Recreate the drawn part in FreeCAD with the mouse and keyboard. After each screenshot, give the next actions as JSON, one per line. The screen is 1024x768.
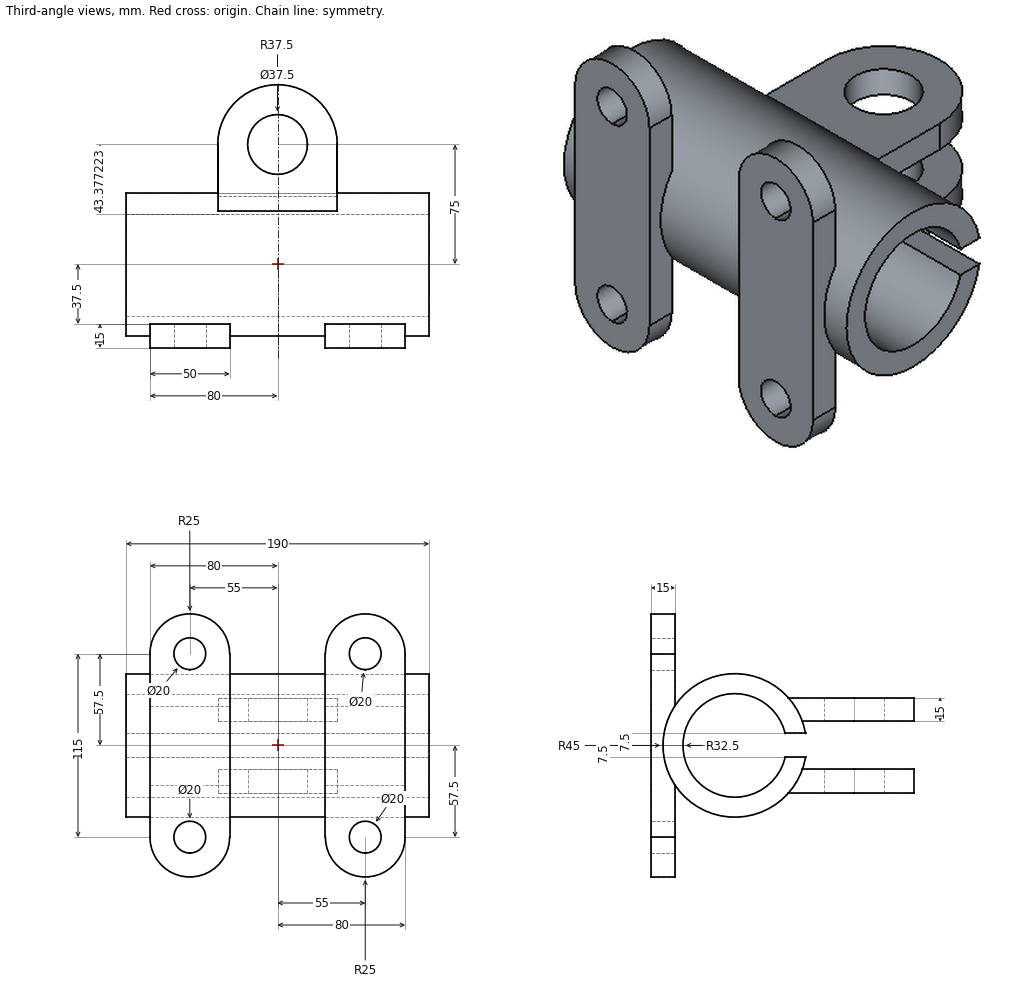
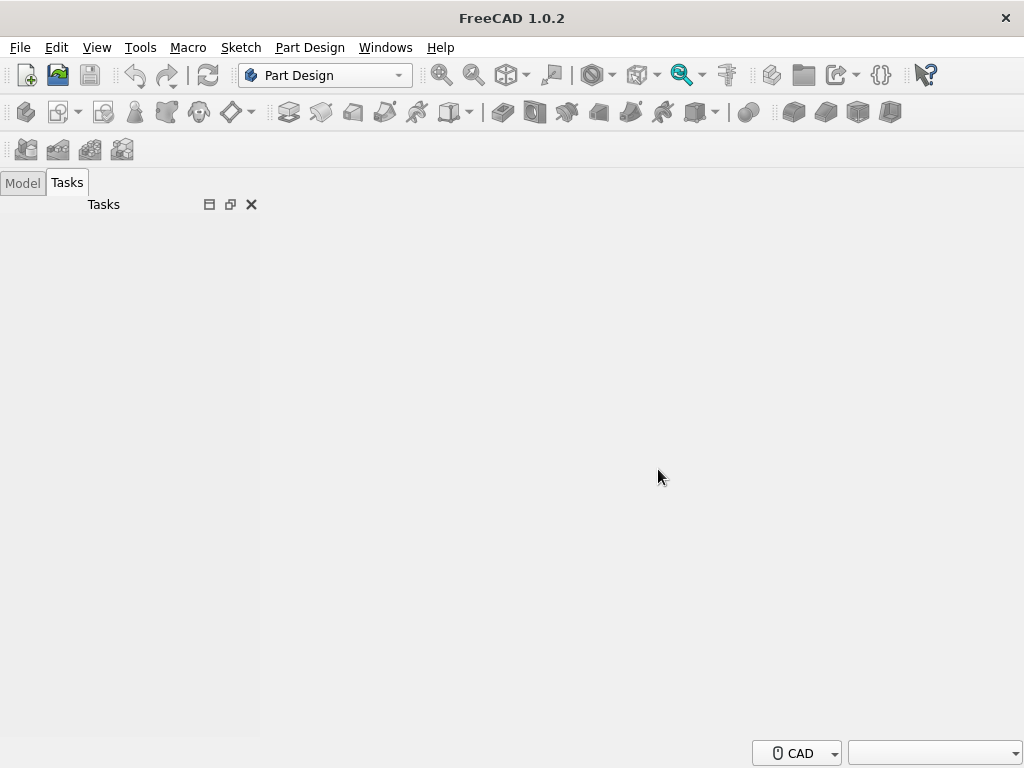
{"action": "left_click", "coordinate": [26, 76]}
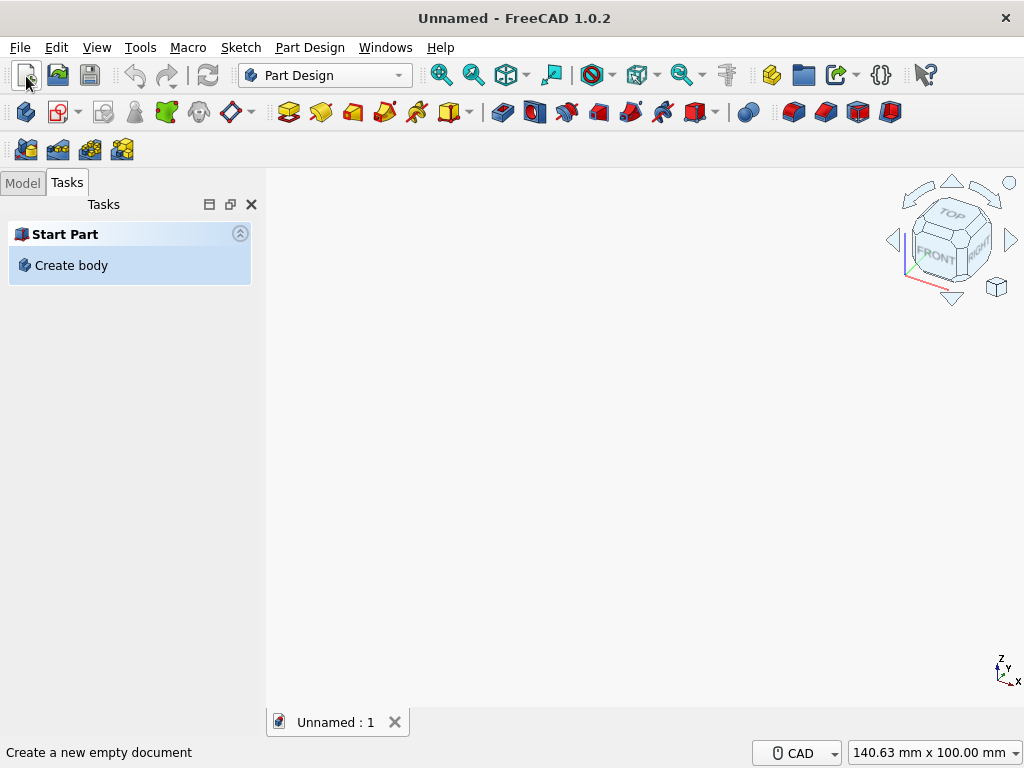
{"action": "left_click", "coordinate": [58, 112]}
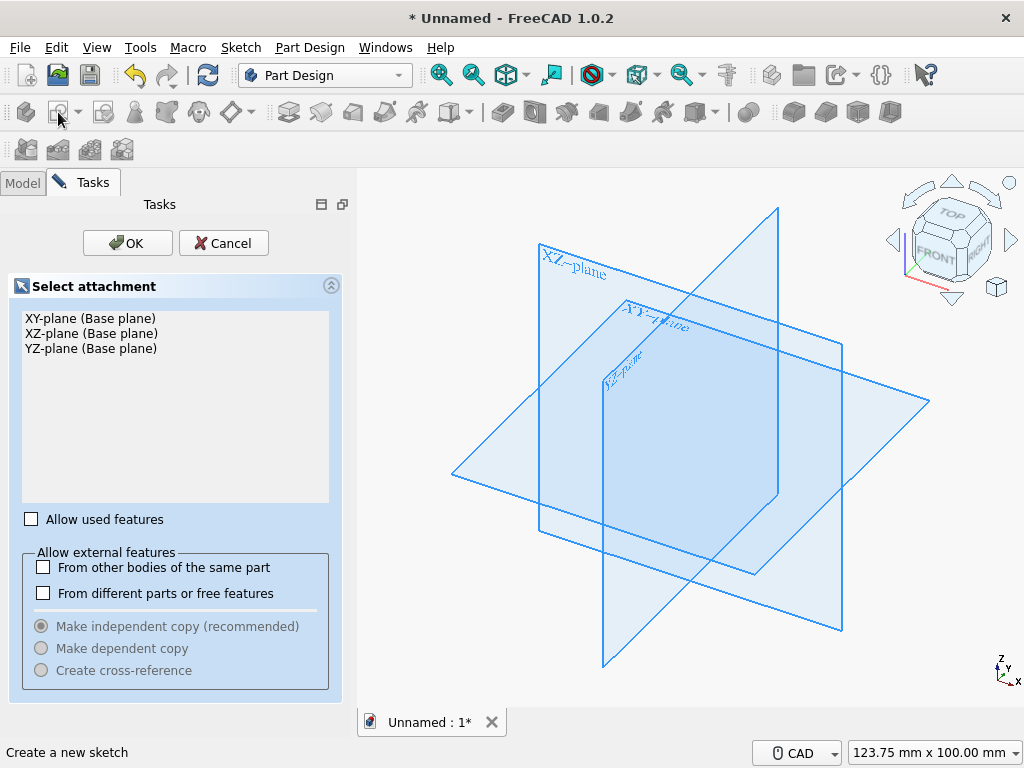
{"action": "left_click", "coordinate": [82, 348]}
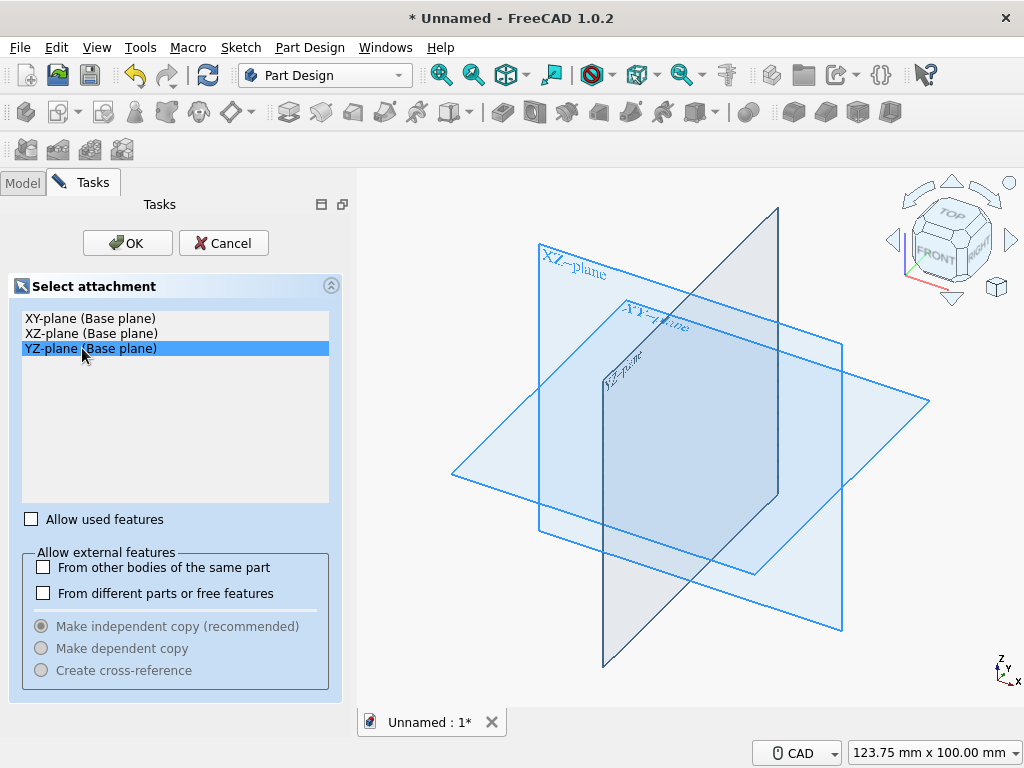
{"action": "left_click", "coordinate": [128, 243]}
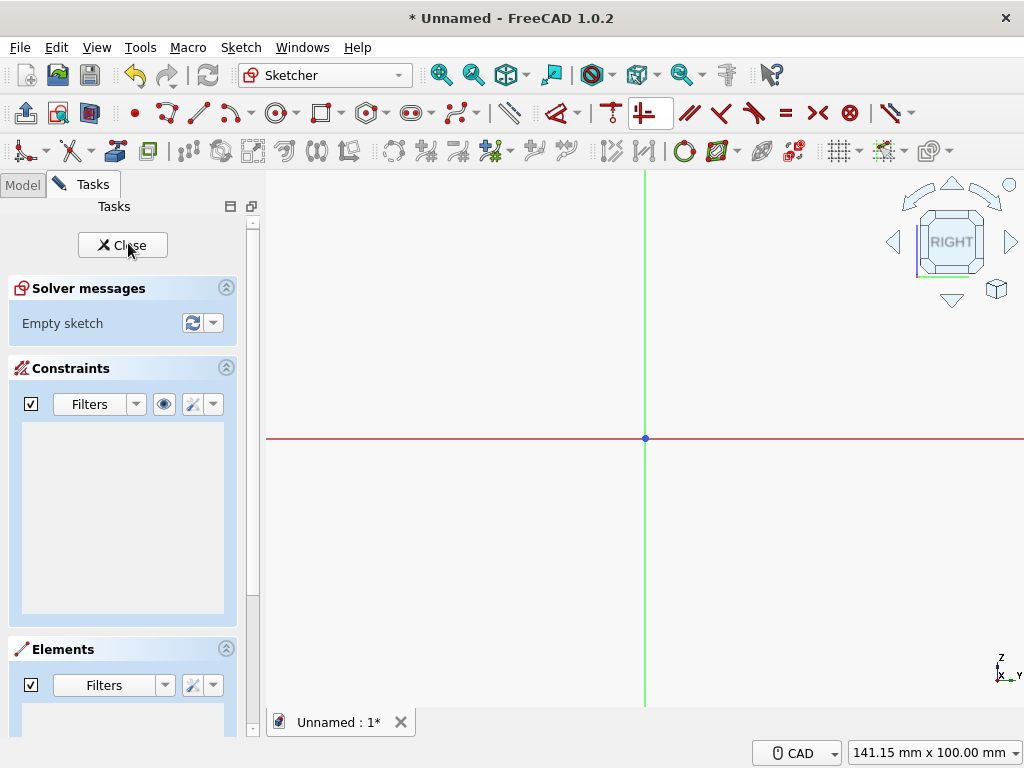
{"action": "scroll", "coordinate": [294, 439], "scroll_direction": "down", "scroll_amount": 1}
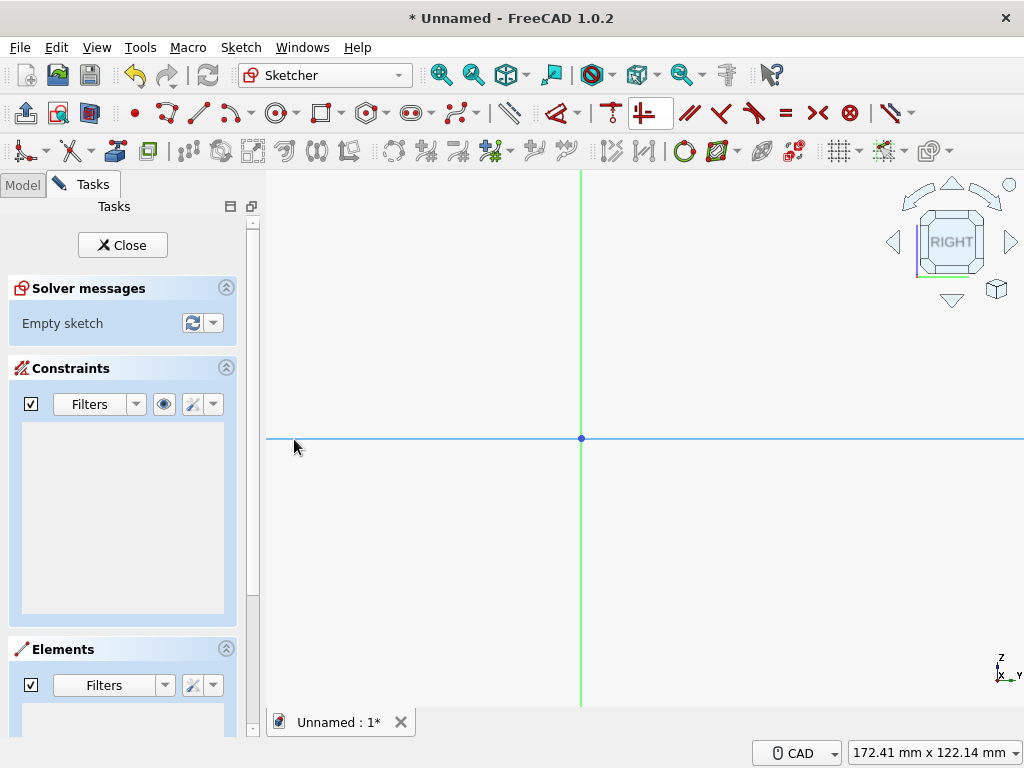
{"action": "left_click", "coordinate": [200, 114]}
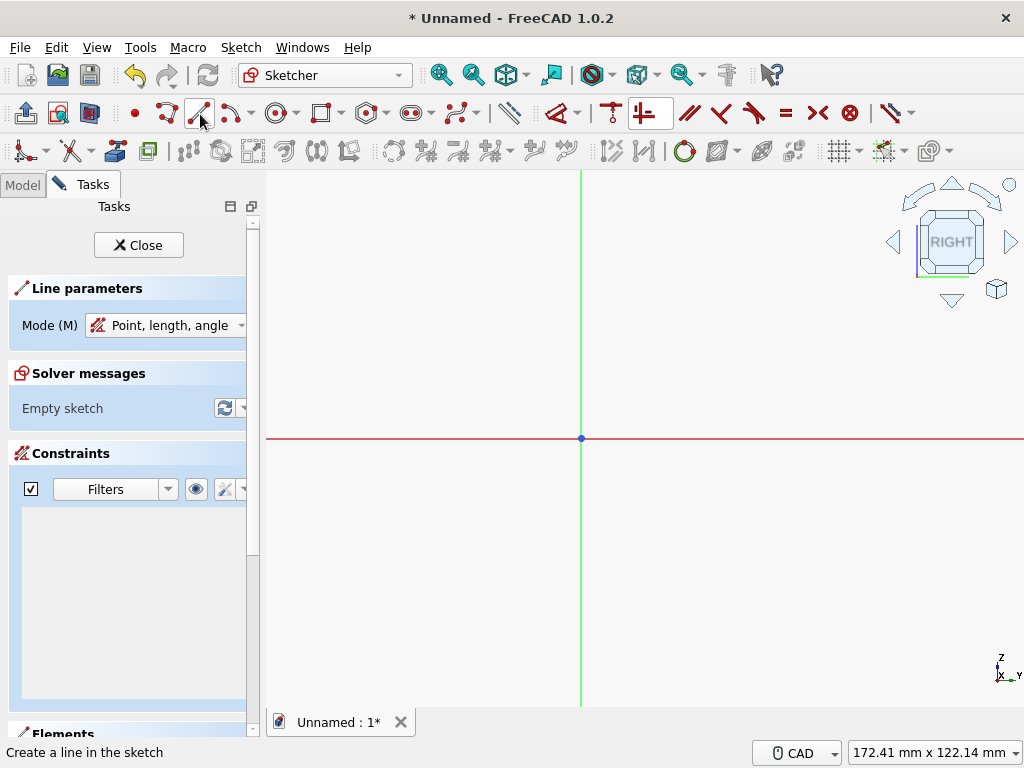
{"action": "left_click", "coordinate": [720, 406]}
{"action": "left_click", "coordinate": [776, 406]}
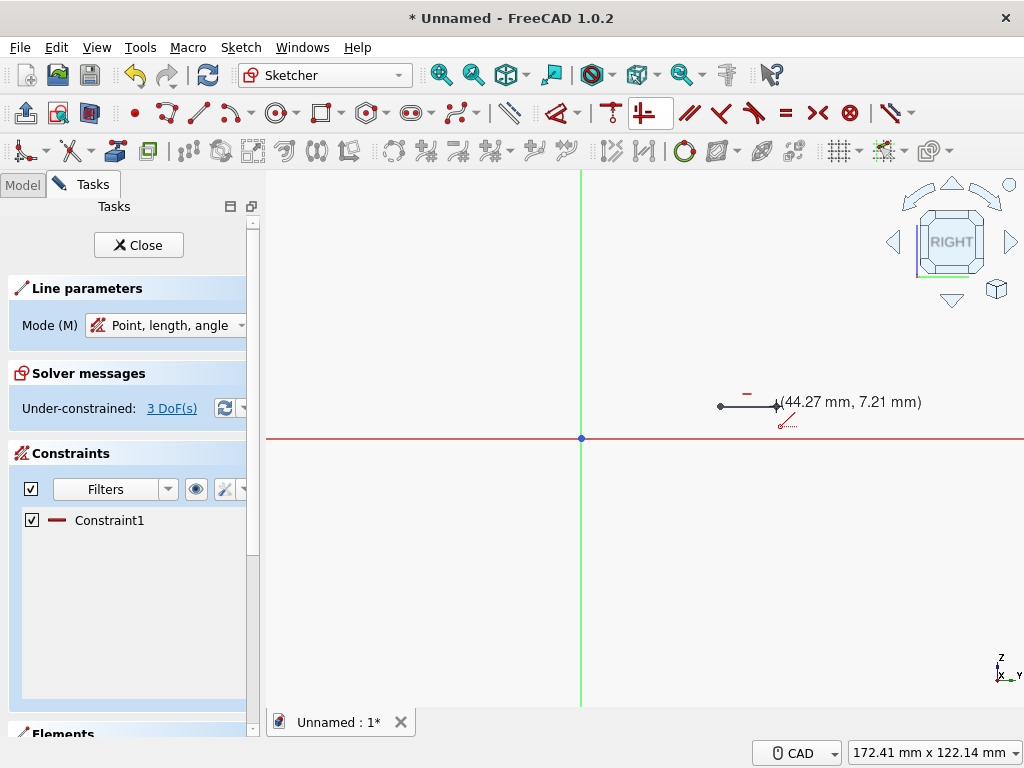
{"action": "left_click", "coordinate": [776, 472]}
{"action": "left_click", "coordinate": [720, 472]}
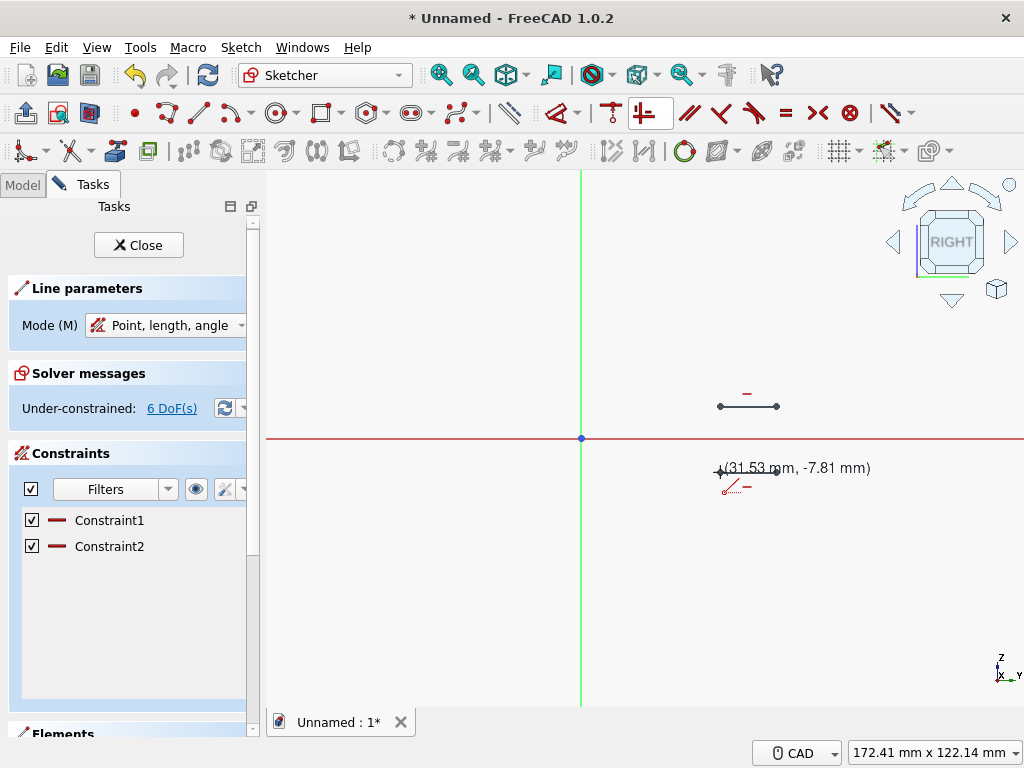
{"action": "left_click", "coordinate": [254, 114]}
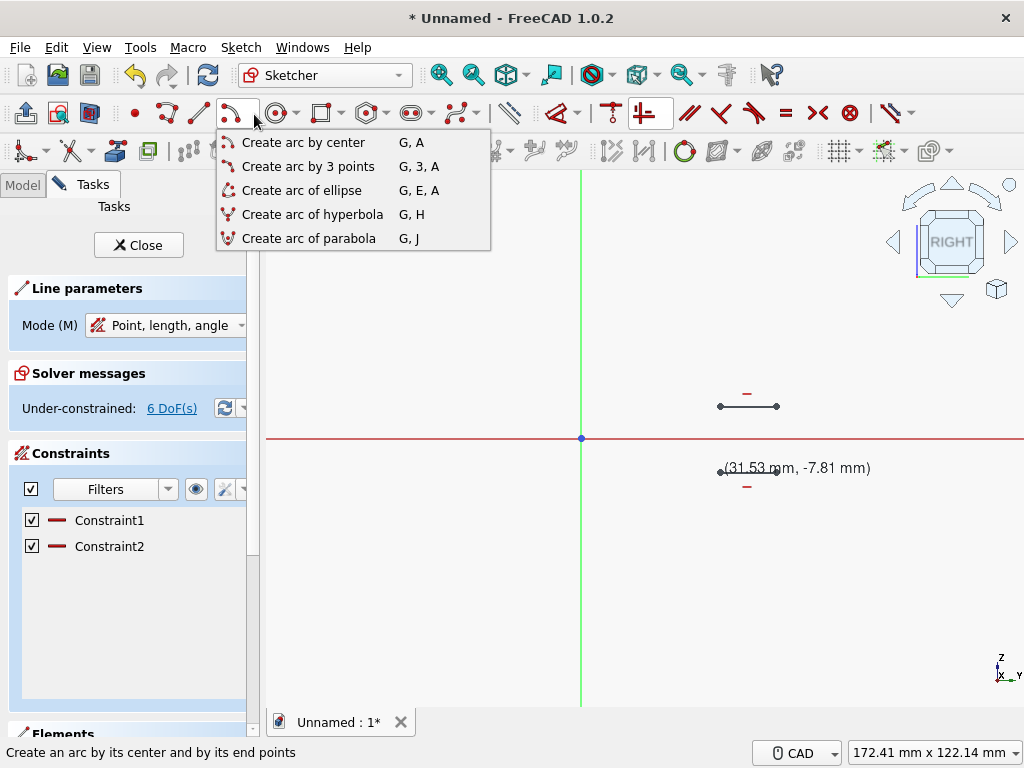
{"action": "left_click", "coordinate": [354, 166]}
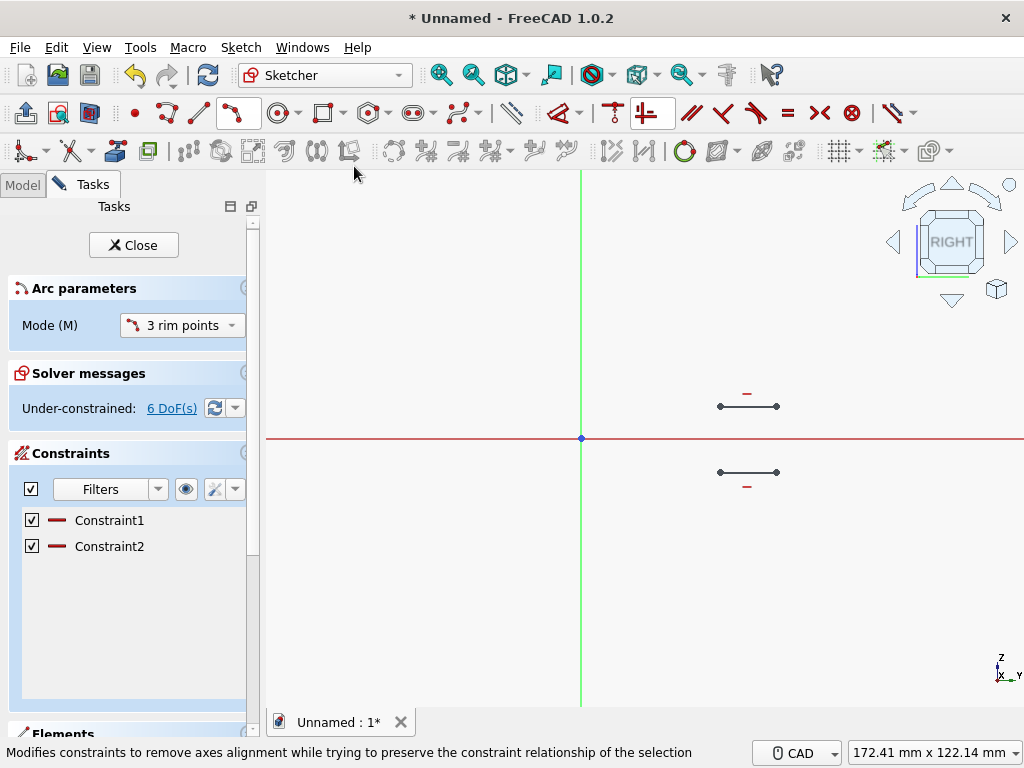
{"action": "left_click", "coordinate": [776, 407]}
{"action": "left_click", "coordinate": [776, 473]}
{"action": "left_click", "coordinate": [418, 328]}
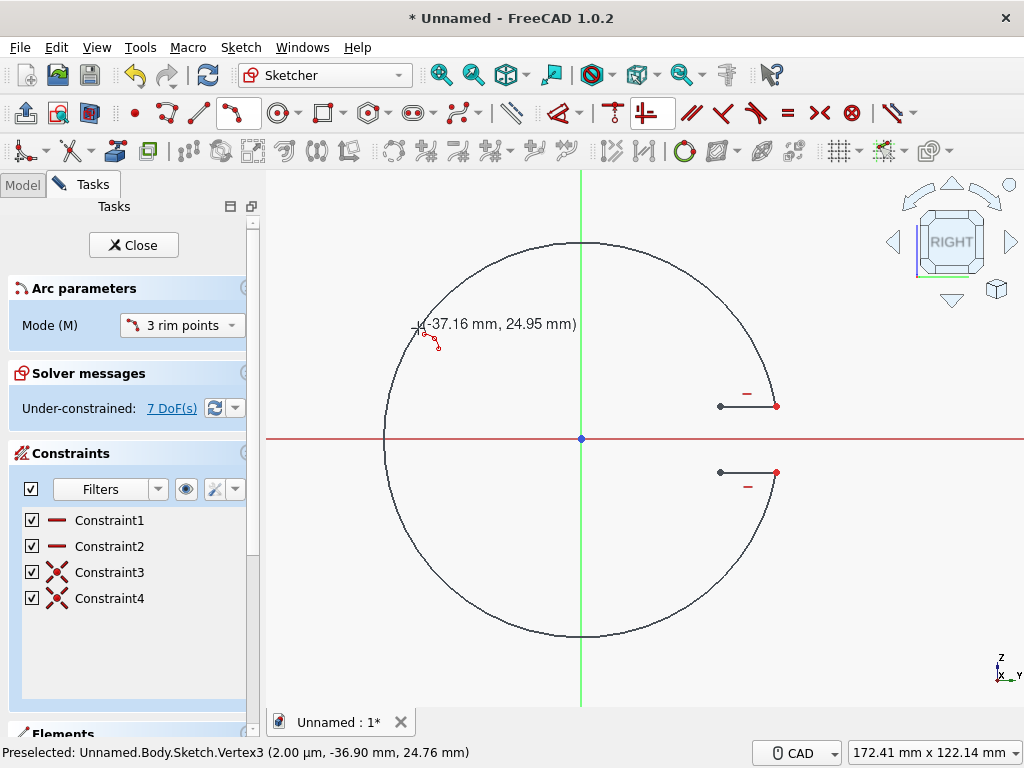
{"action": "left_click", "coordinate": [720, 473]}
{"action": "left_click", "coordinate": [720, 407]}
{"action": "left_click", "coordinate": [462, 360]}
{"action": "key", "text": "Escape"}